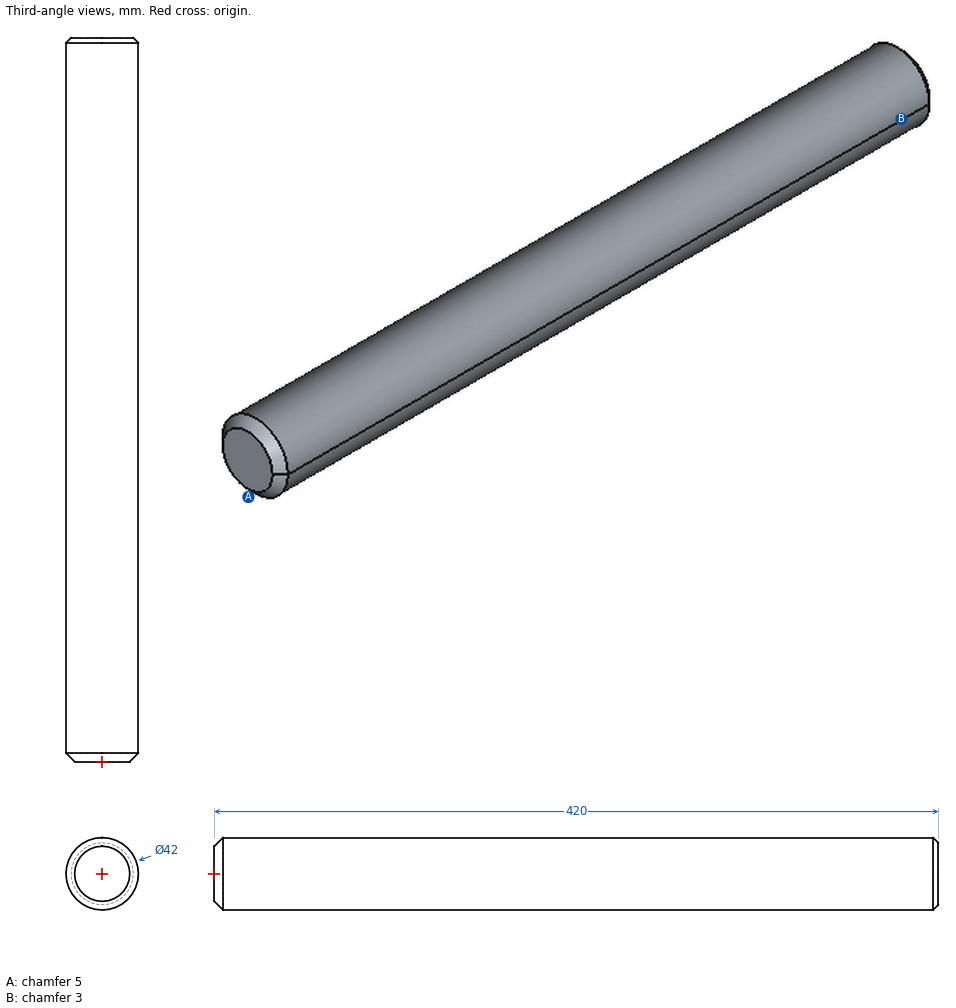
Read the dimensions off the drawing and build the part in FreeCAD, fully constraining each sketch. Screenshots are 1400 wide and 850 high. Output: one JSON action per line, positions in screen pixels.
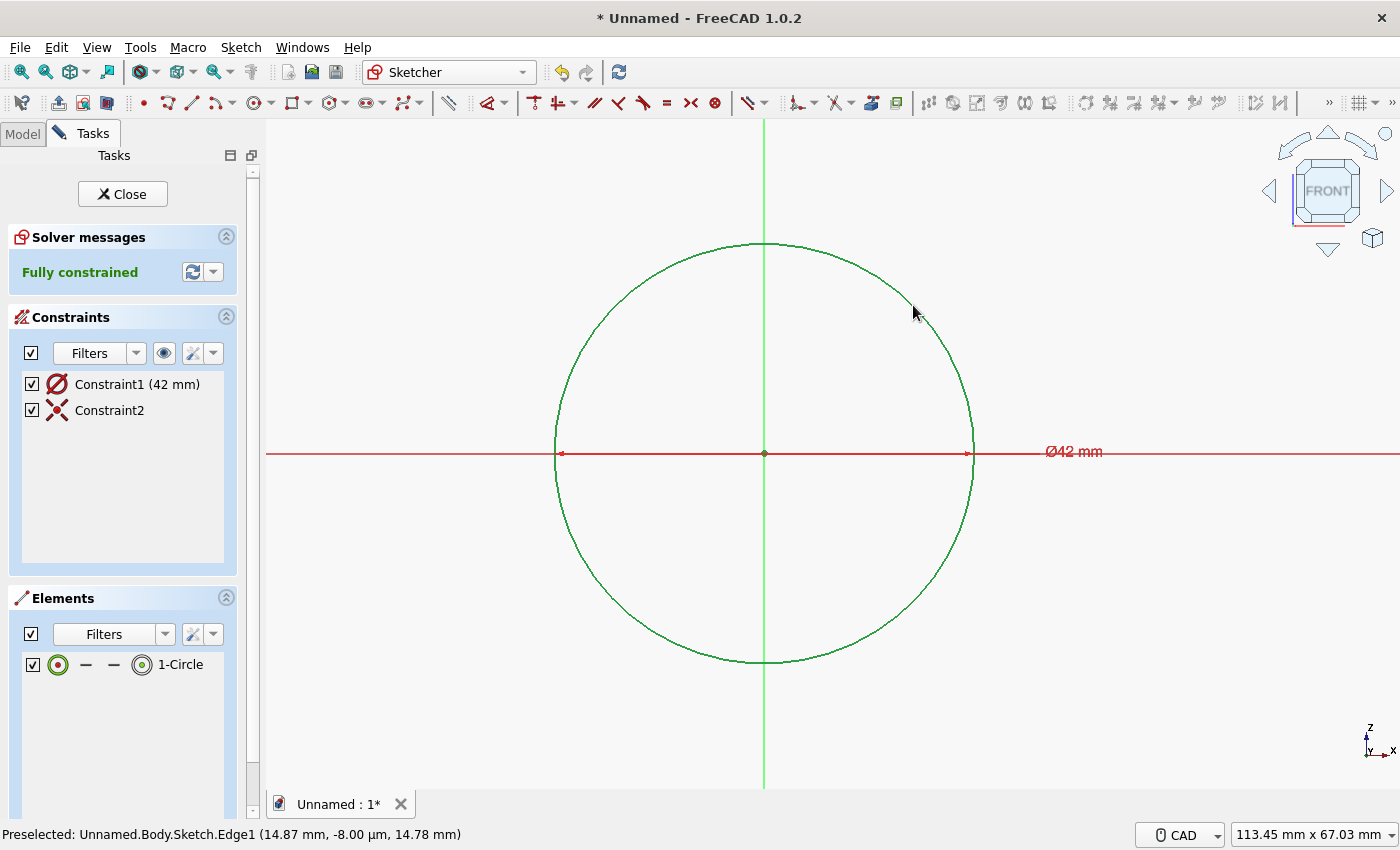
{"action": "left_click", "coordinate": [123, 194]}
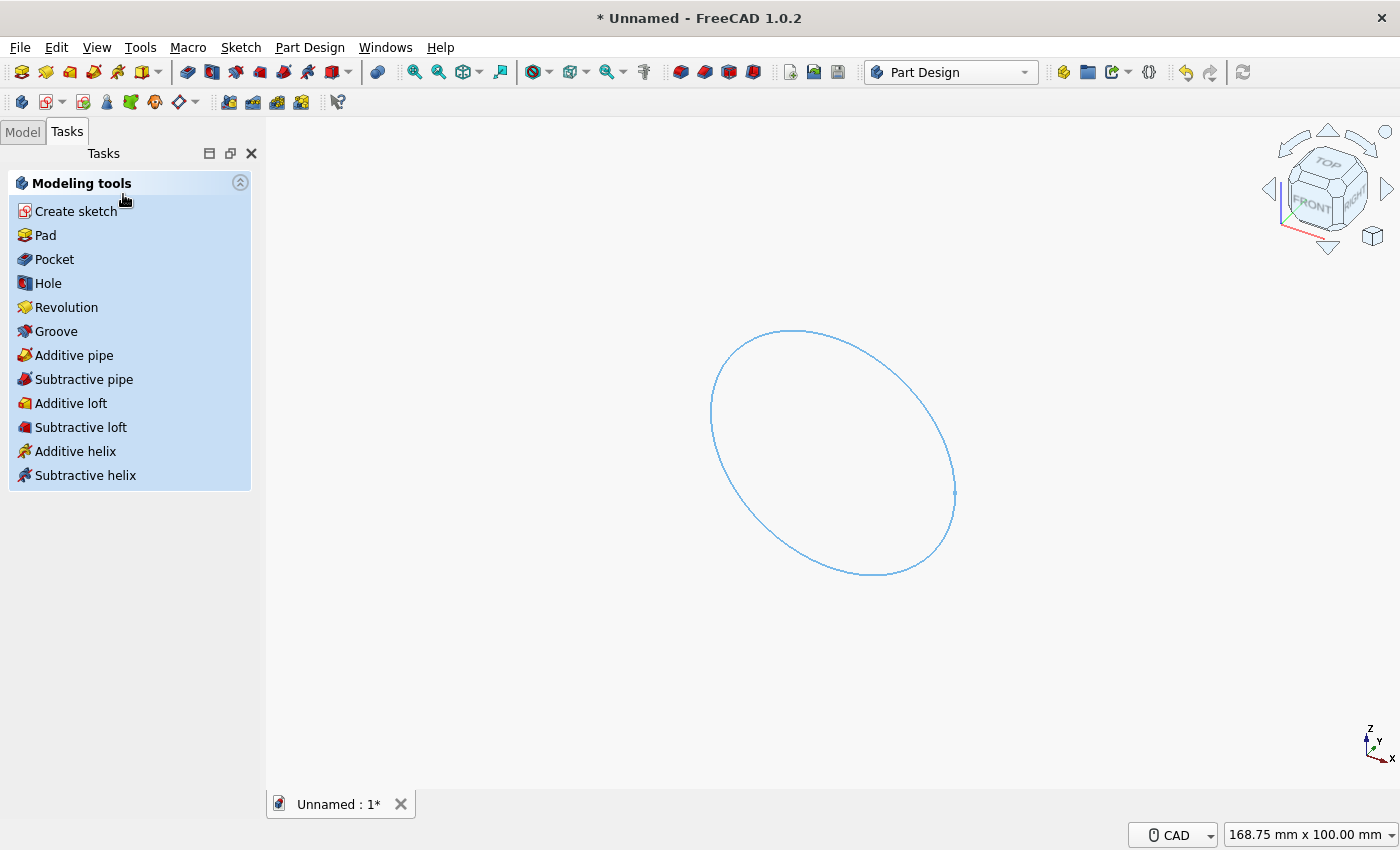
{"action": "left_click", "coordinate": [22, 72]}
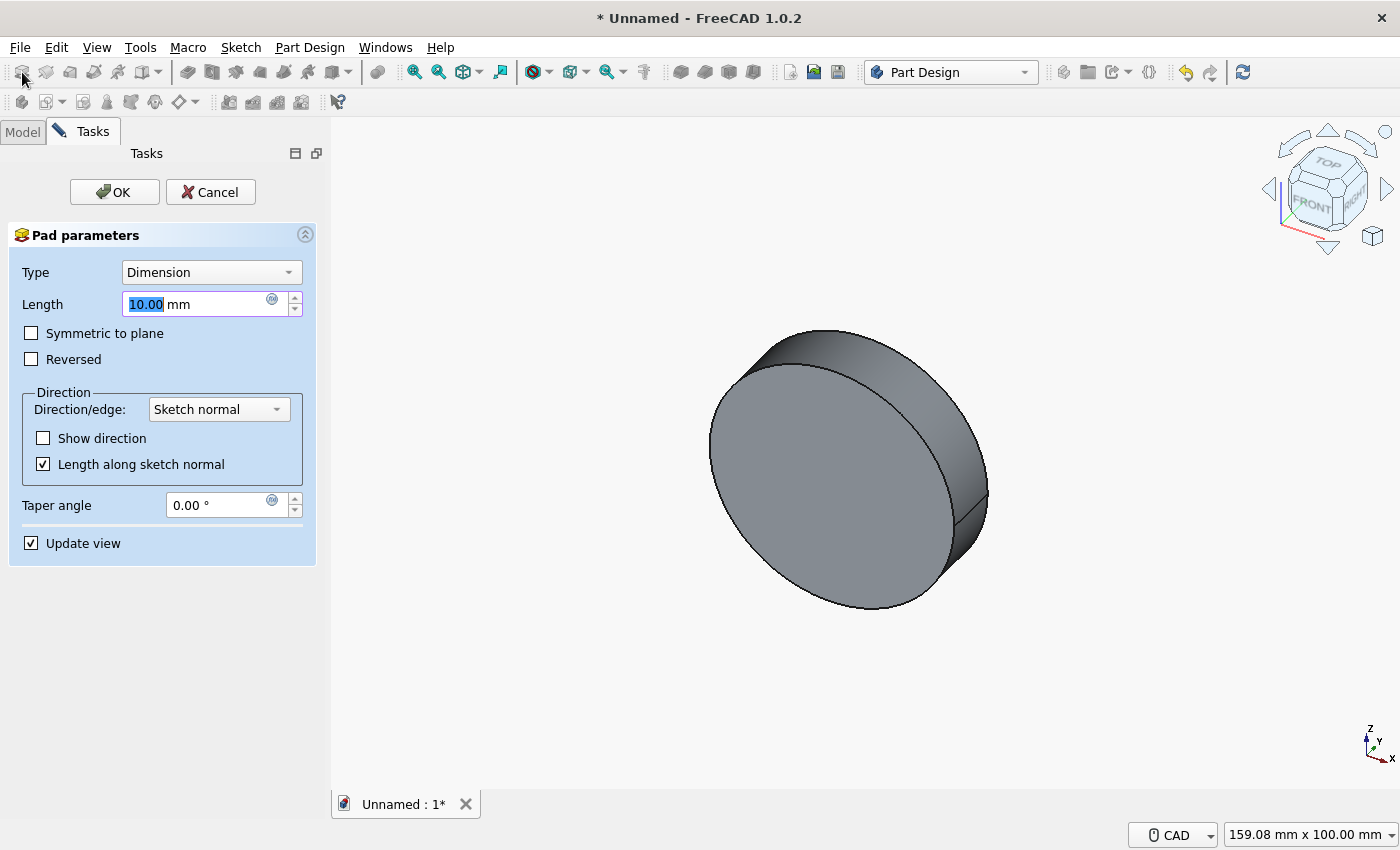
{"action": "type", "text": "420"}
{"action": "key", "text": "Tab"}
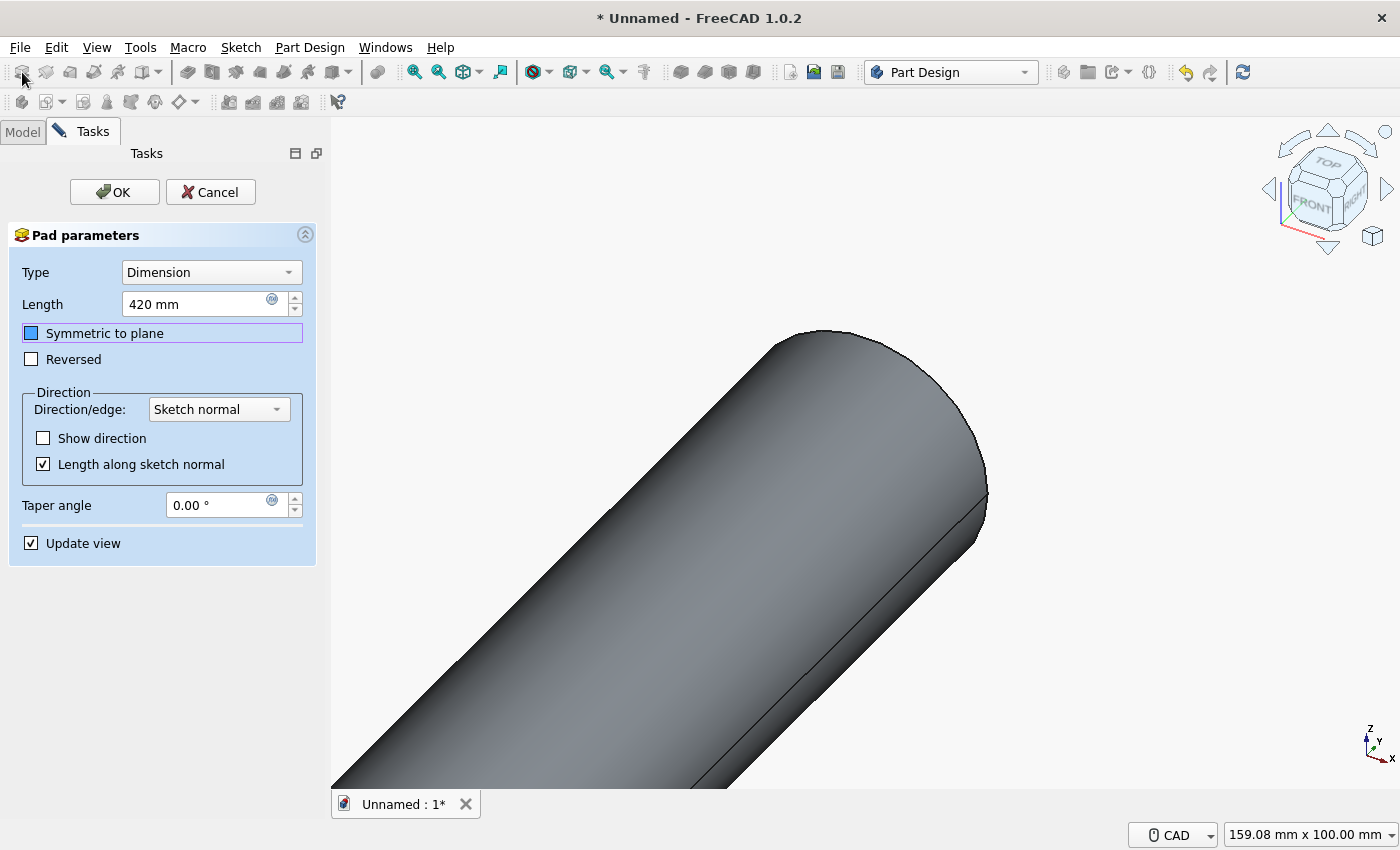
{"action": "left_click", "coordinate": [30, 359]}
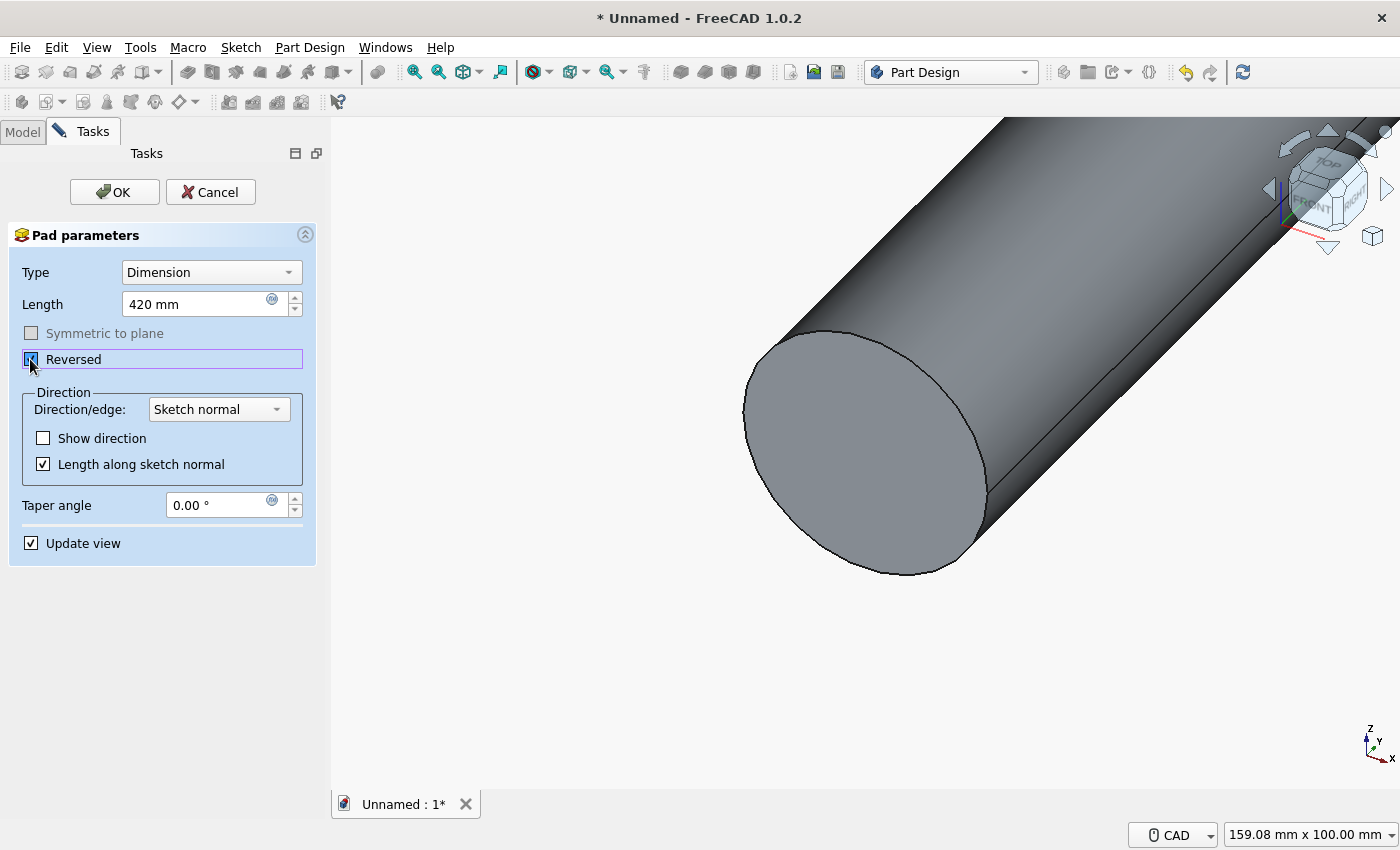
{"action": "left_click", "coordinate": [115, 192]}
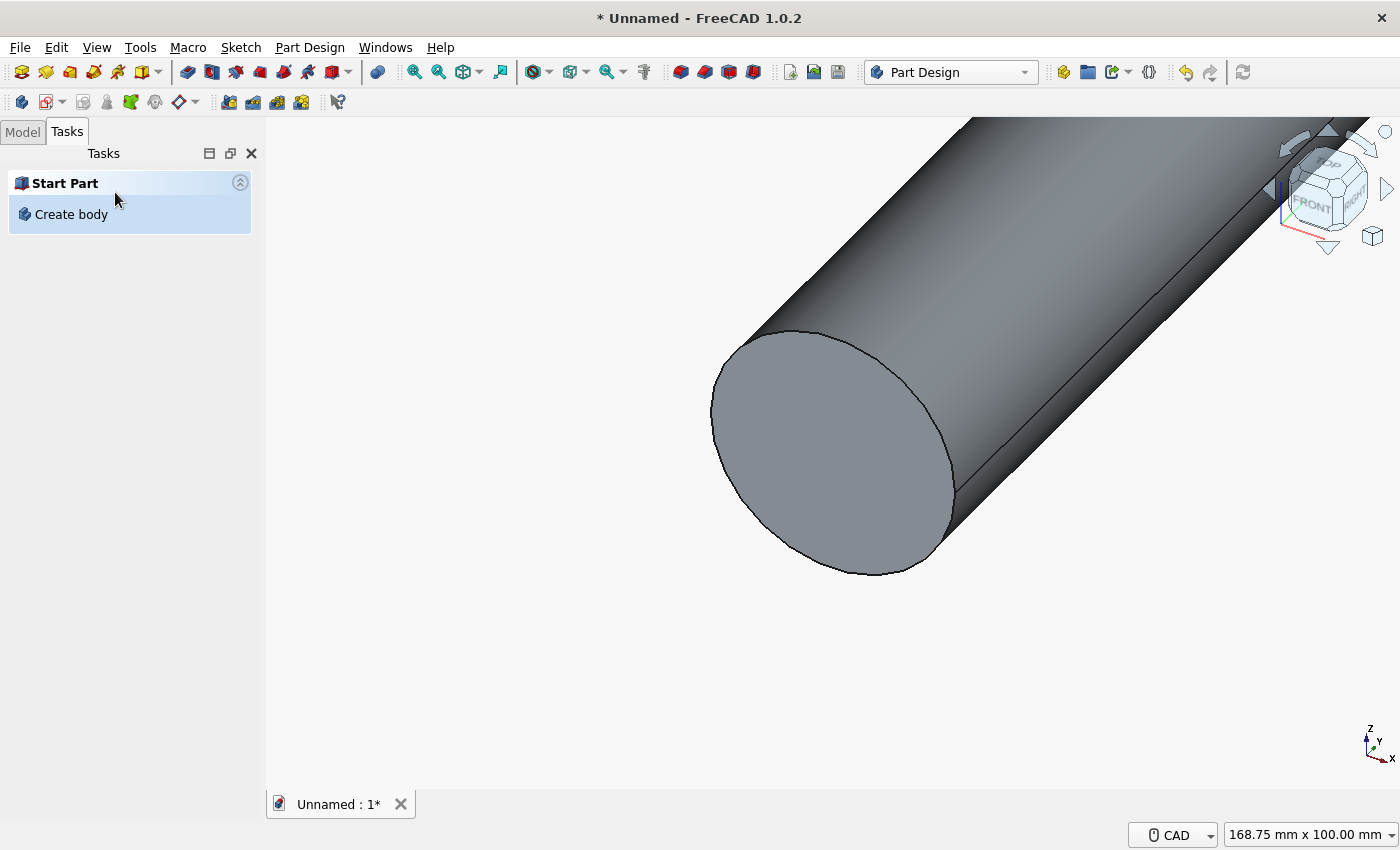
{"action": "key", "text": "v f"}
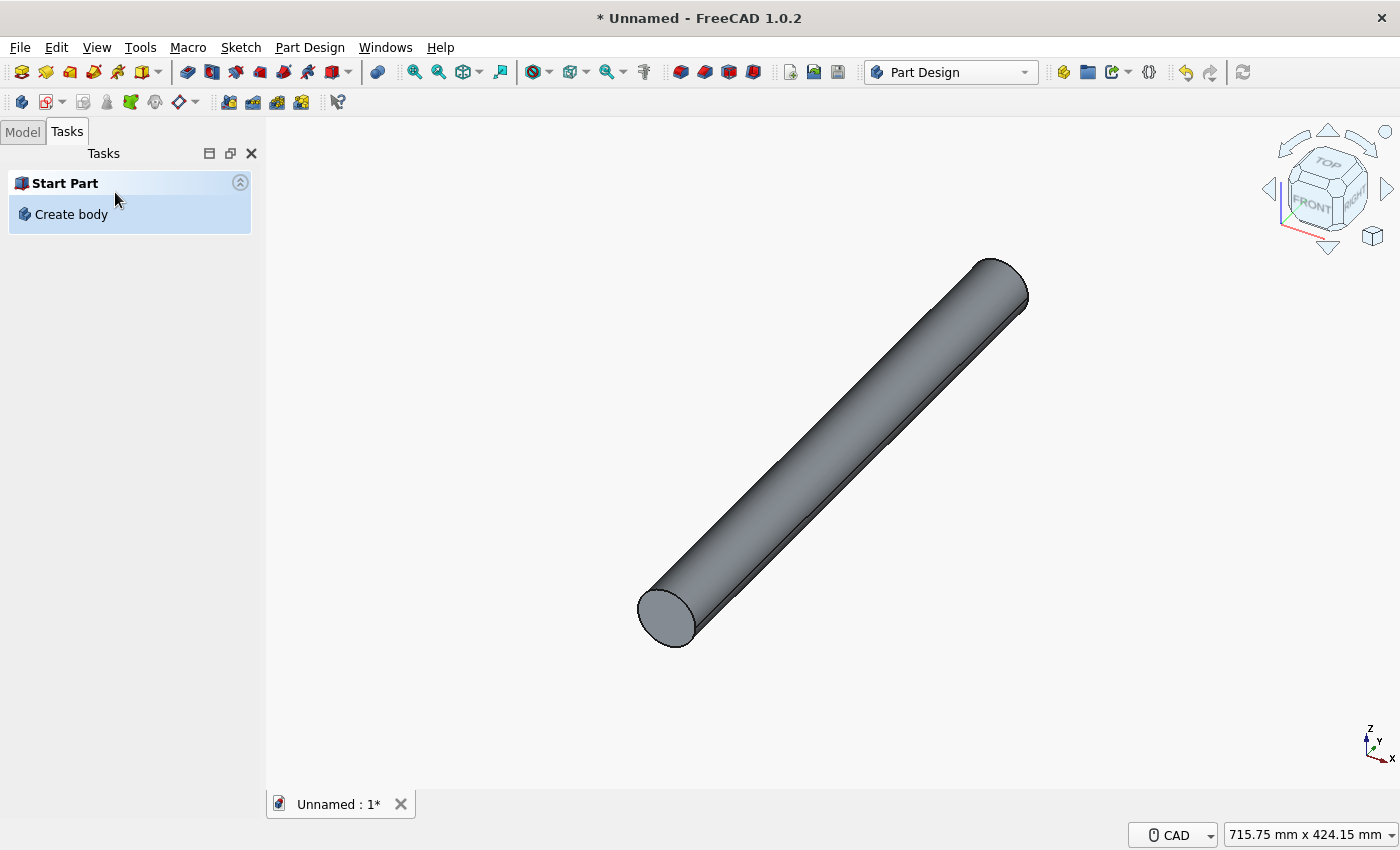
{"action": "left_click", "coordinate": [643, 594]}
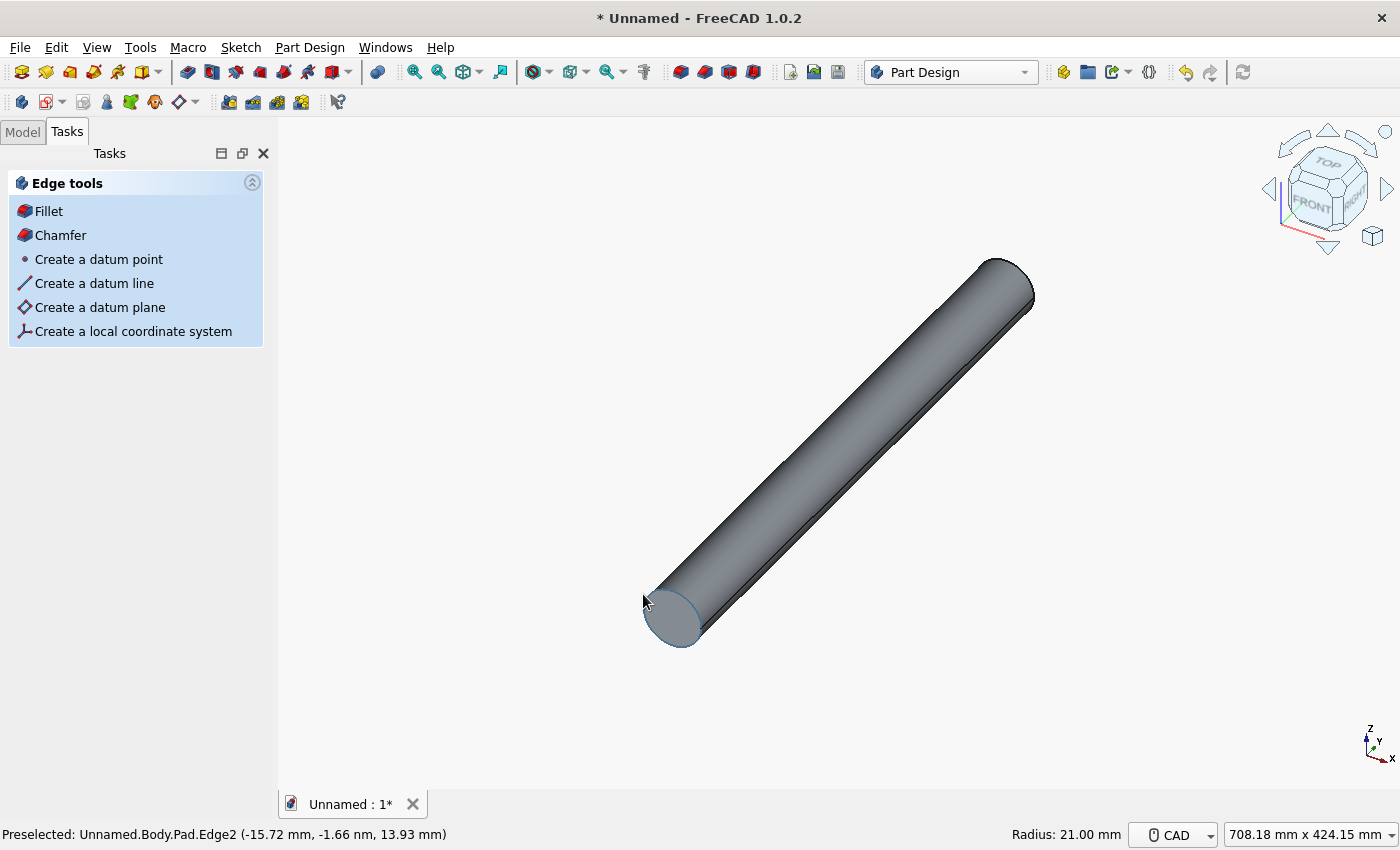
{"action": "left_click", "coordinate": [706, 72]}